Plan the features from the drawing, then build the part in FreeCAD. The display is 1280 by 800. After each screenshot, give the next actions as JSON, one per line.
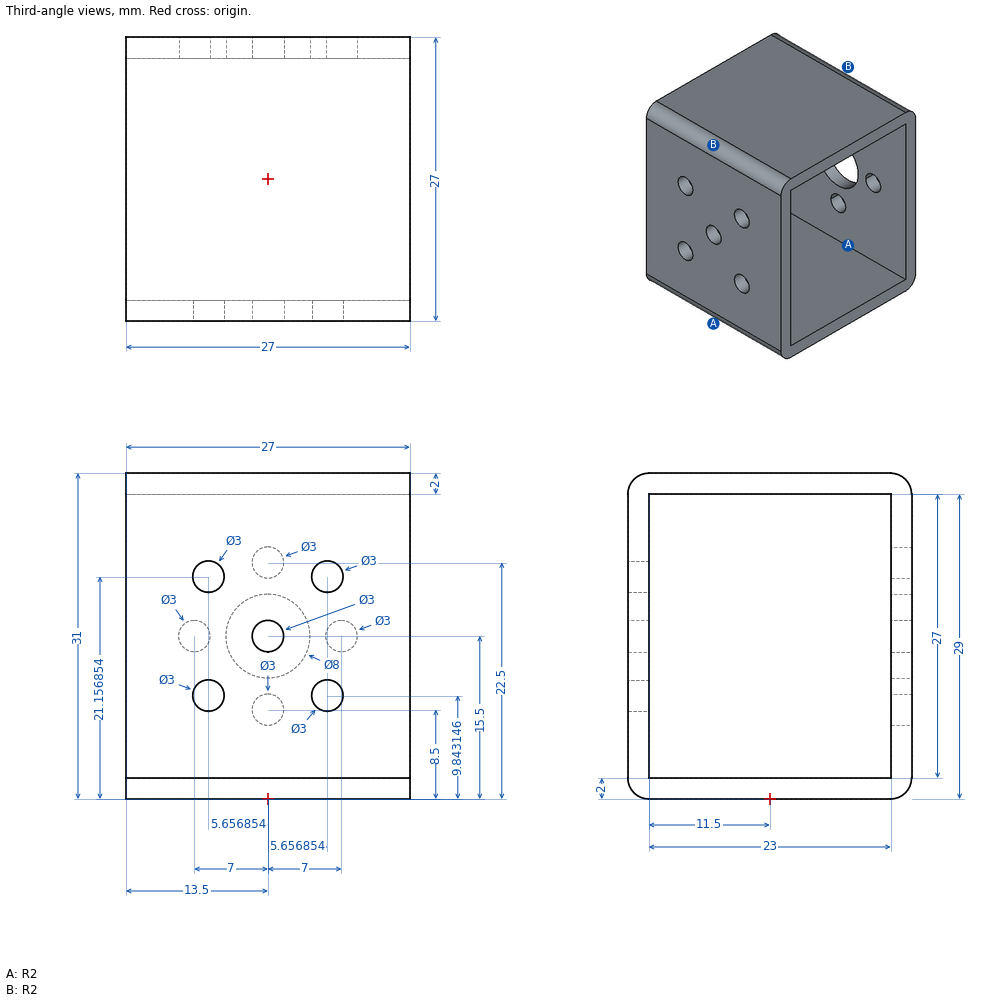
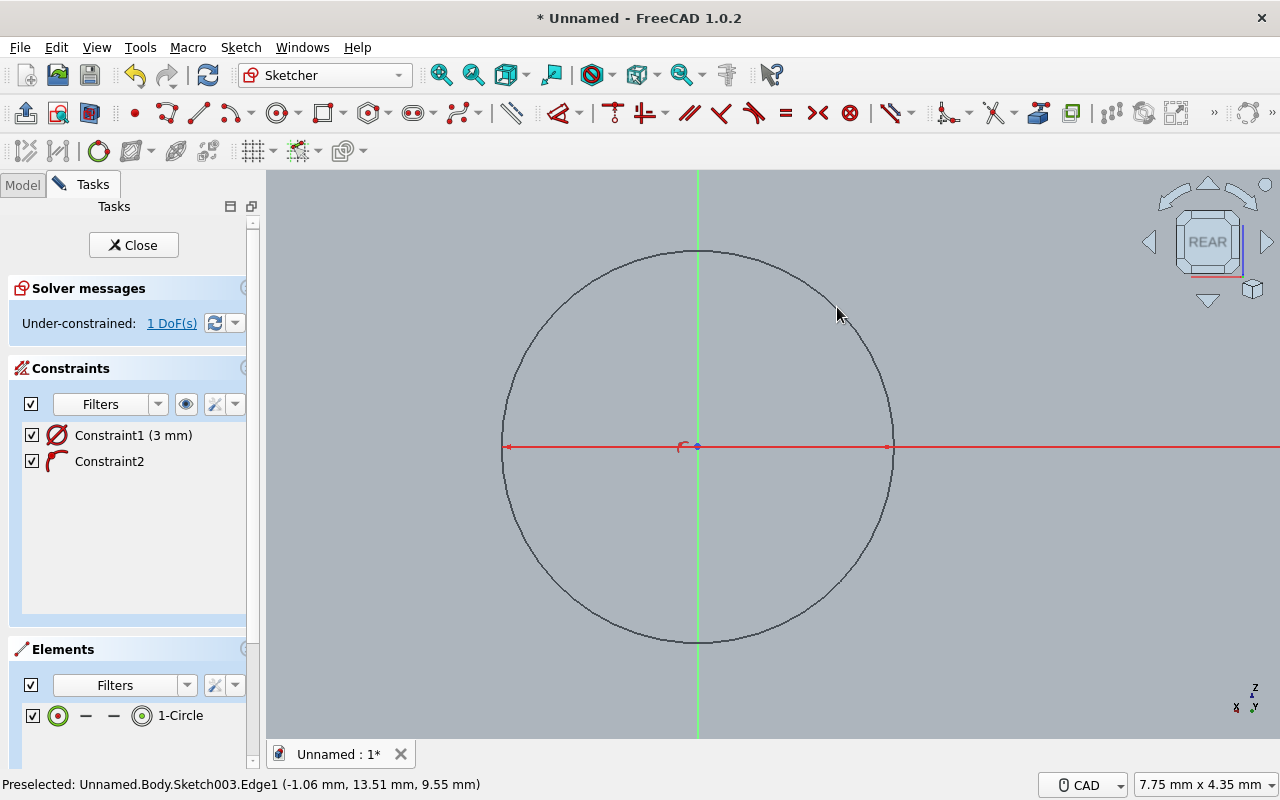
{"action": "left_click", "coordinate": [558, 114]}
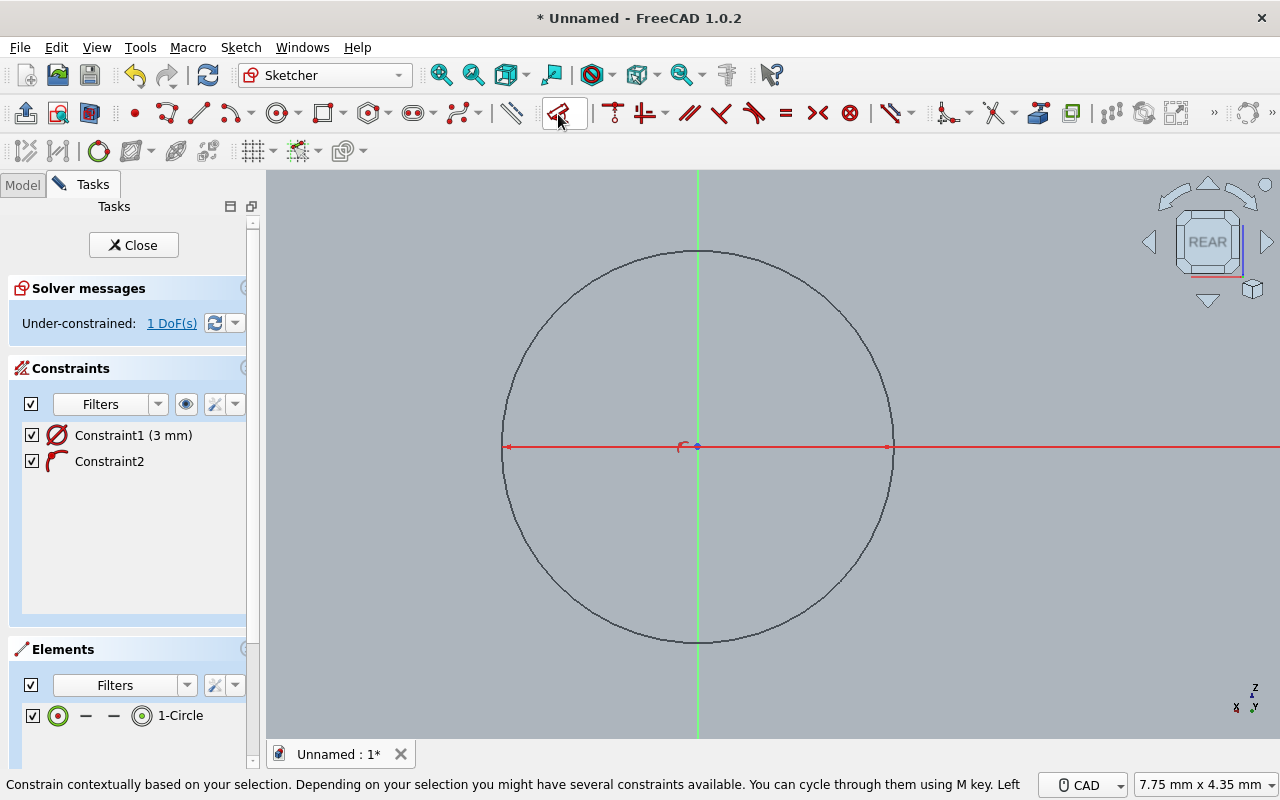
{"action": "left_click", "coordinate": [698, 447]}
{"action": "left_click", "coordinate": [732, 579]}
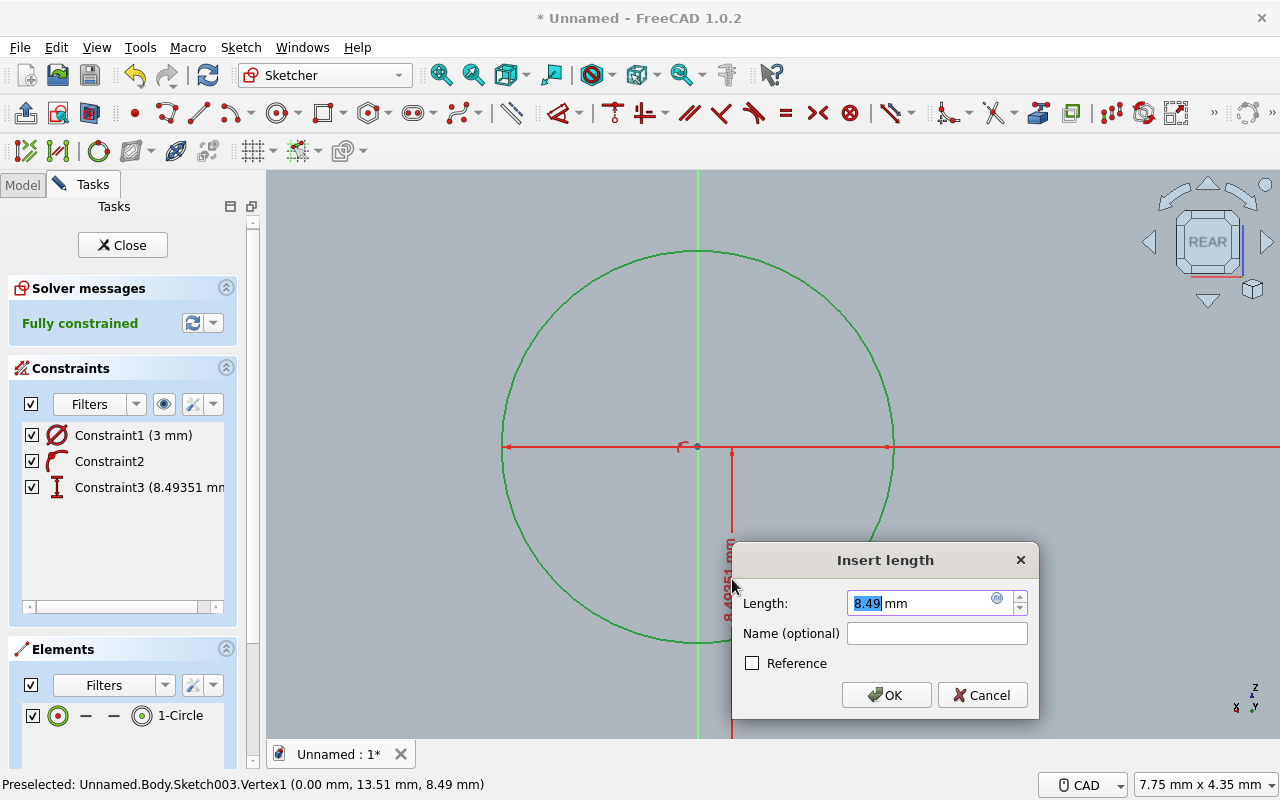
{"action": "type", "text": "8.5"}
{"action": "key", "text": "Return"}
{"action": "key", "text": "Escape"}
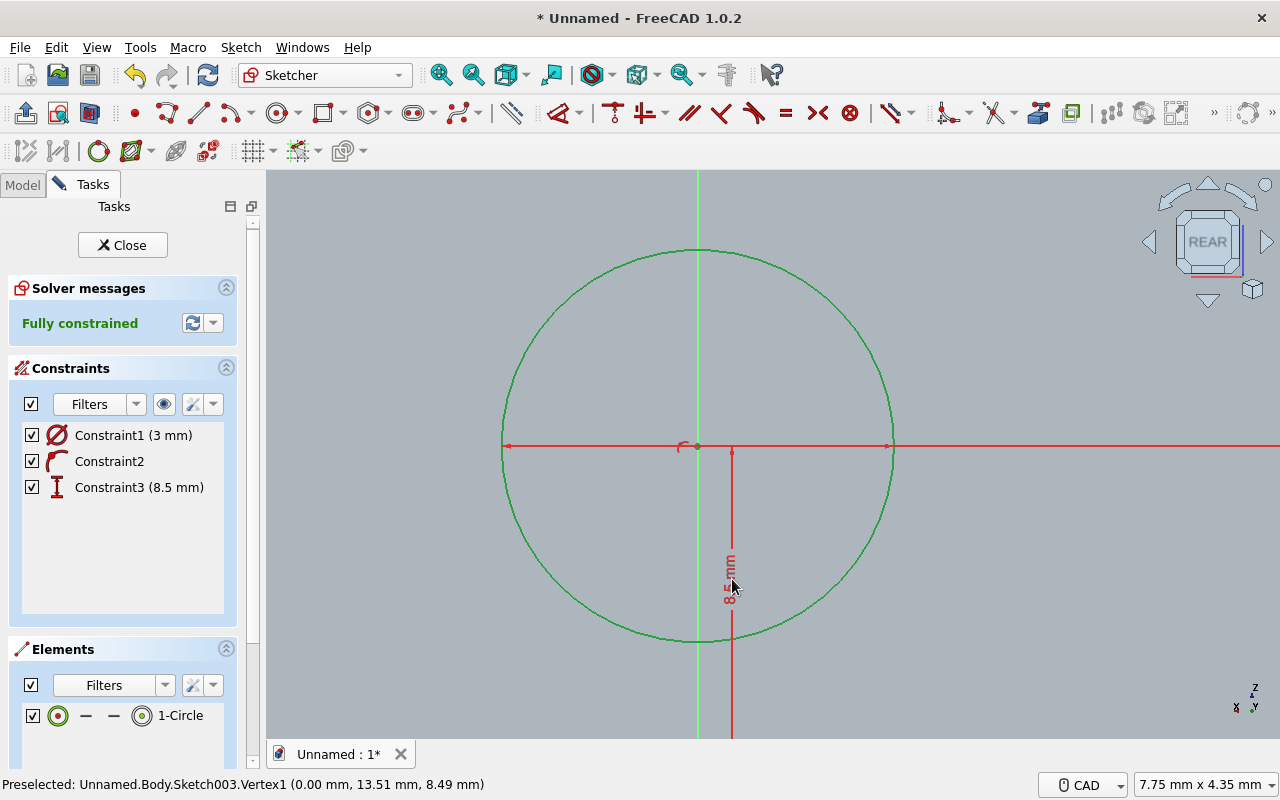
{"action": "left_click", "coordinate": [123, 245]}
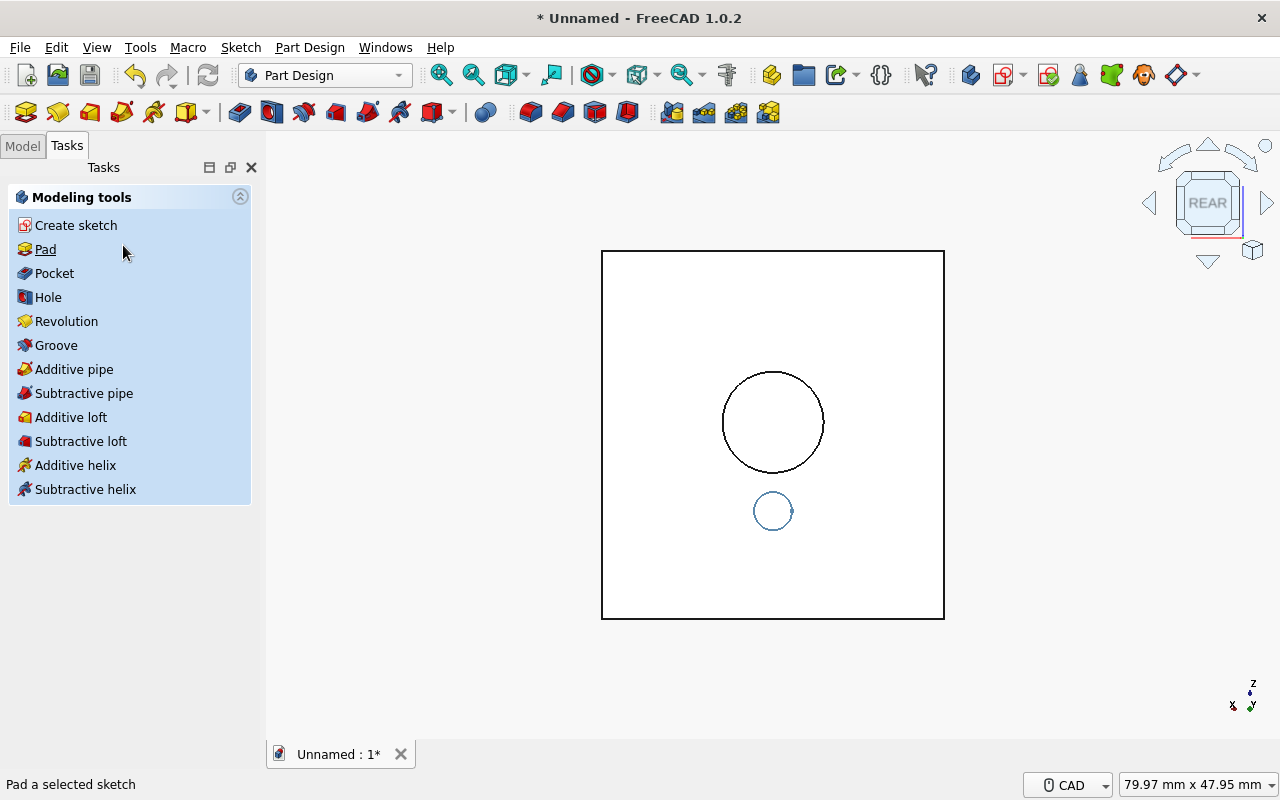
{"action": "left_click", "coordinate": [240, 112]}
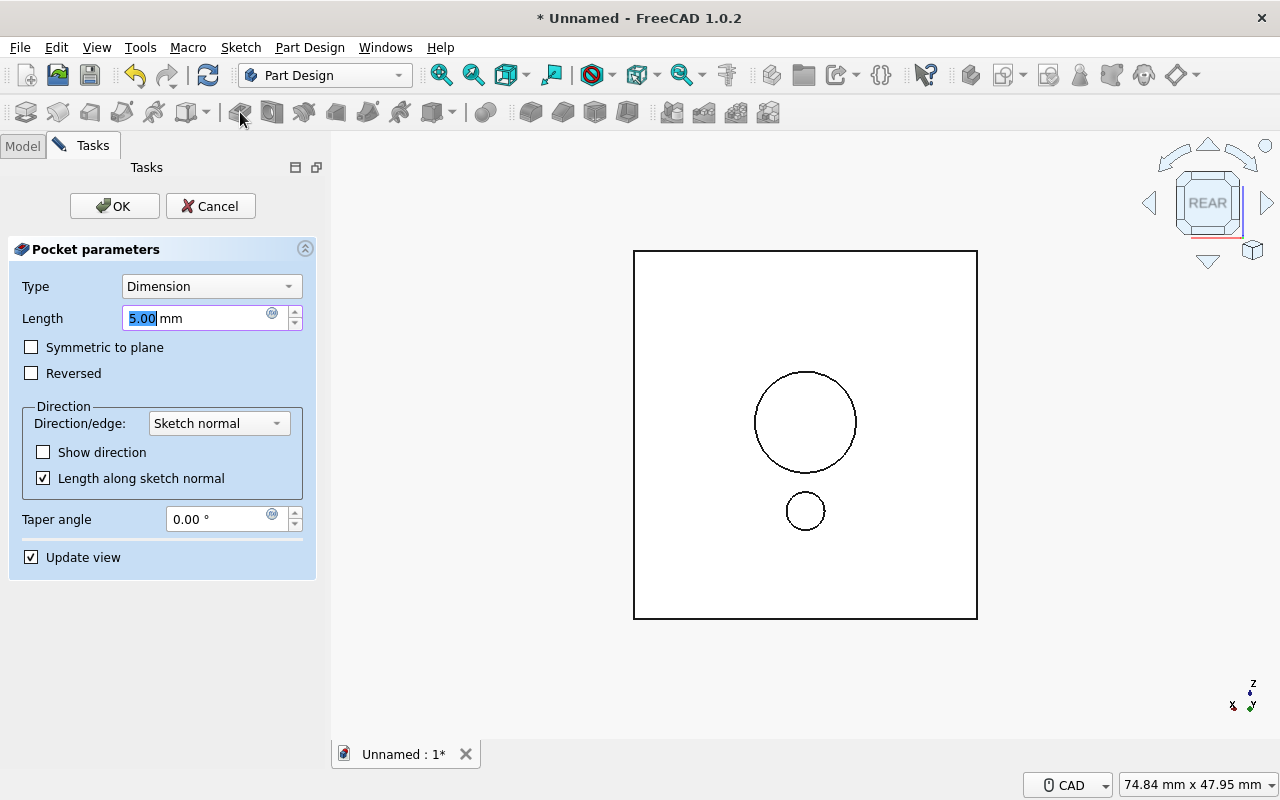
{"action": "left_click", "coordinate": [212, 286]}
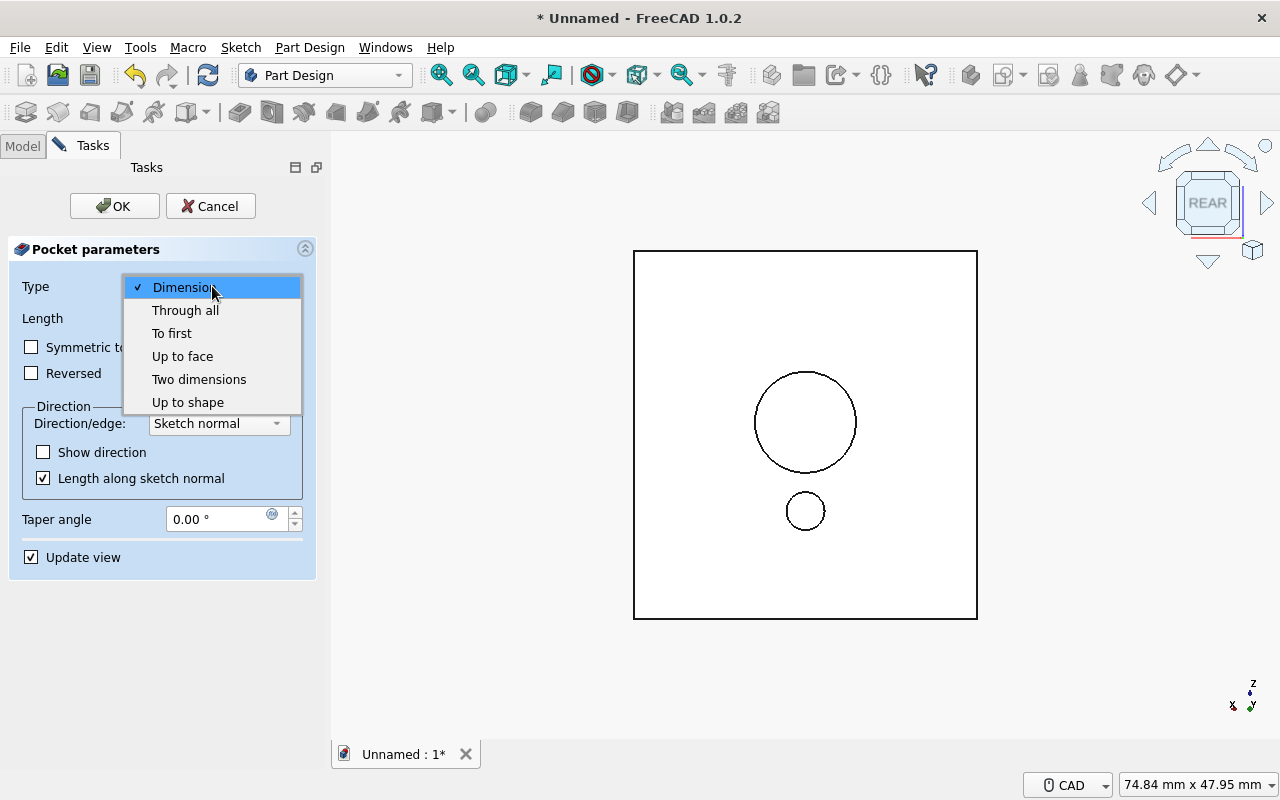
{"action": "left_click", "coordinate": [212, 334]}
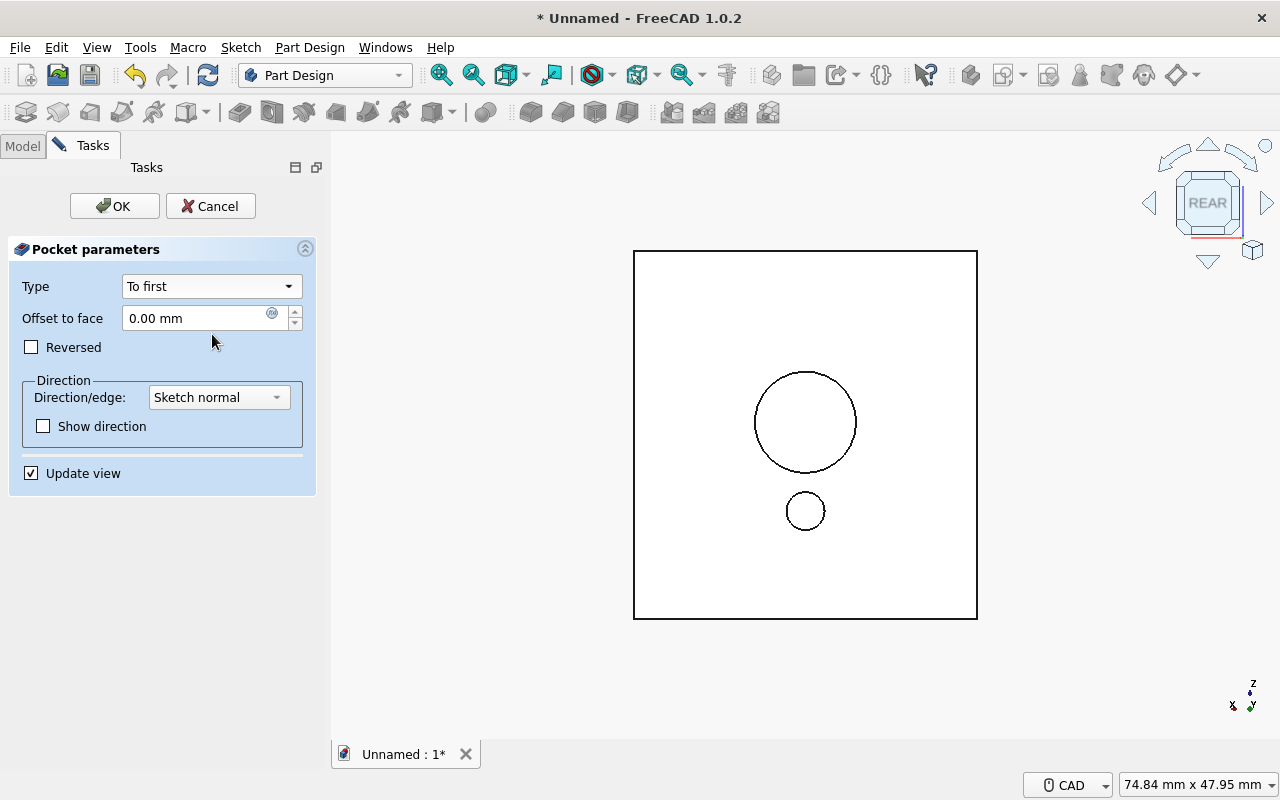
{"action": "left_click", "coordinate": [115, 206]}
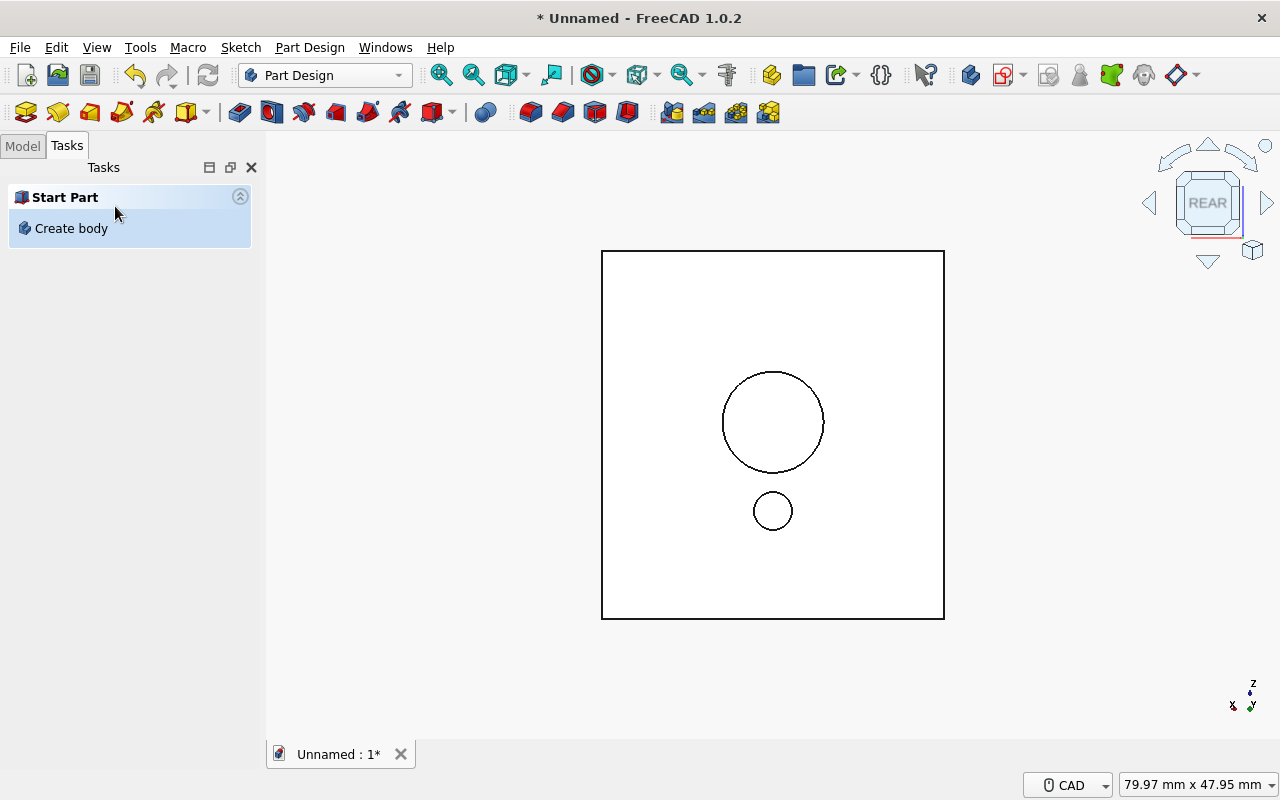
{"action": "left_click", "coordinate": [675, 329]}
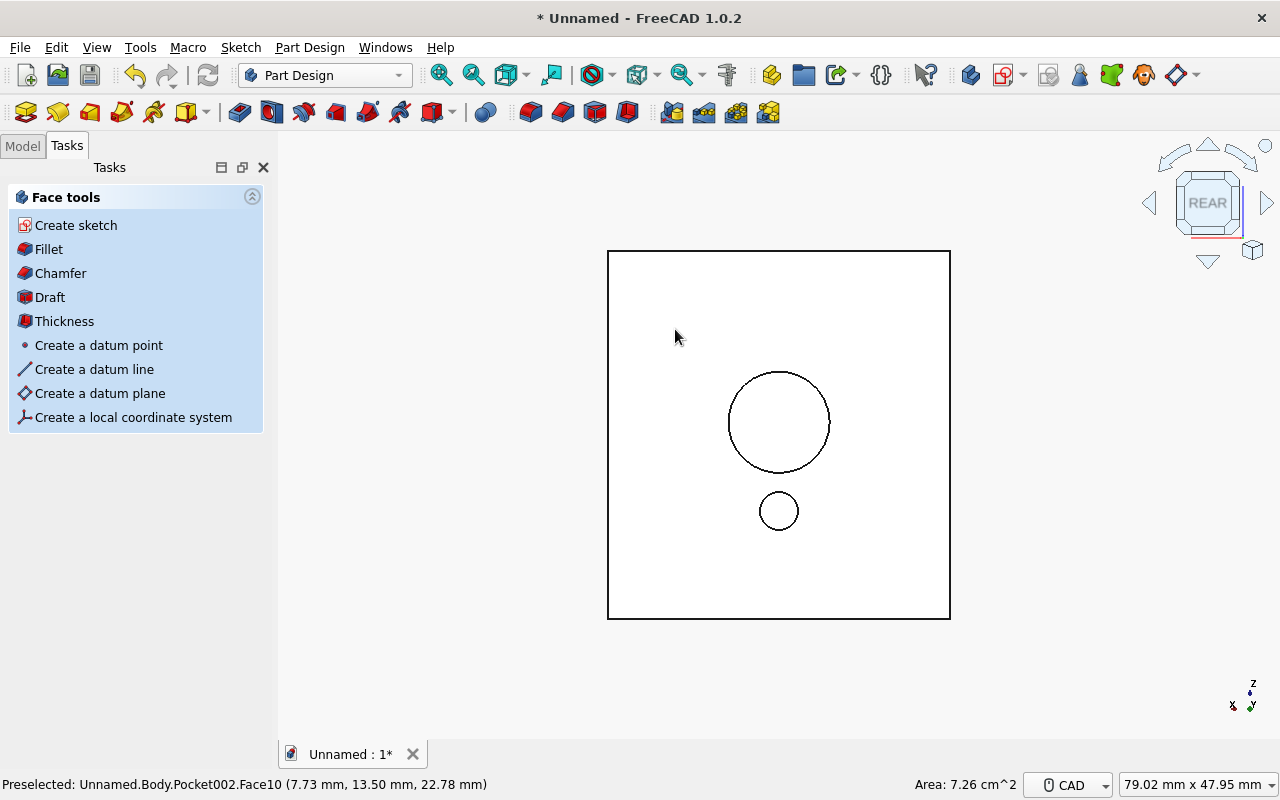
{"action": "left_click", "coordinate": [1004, 76]}